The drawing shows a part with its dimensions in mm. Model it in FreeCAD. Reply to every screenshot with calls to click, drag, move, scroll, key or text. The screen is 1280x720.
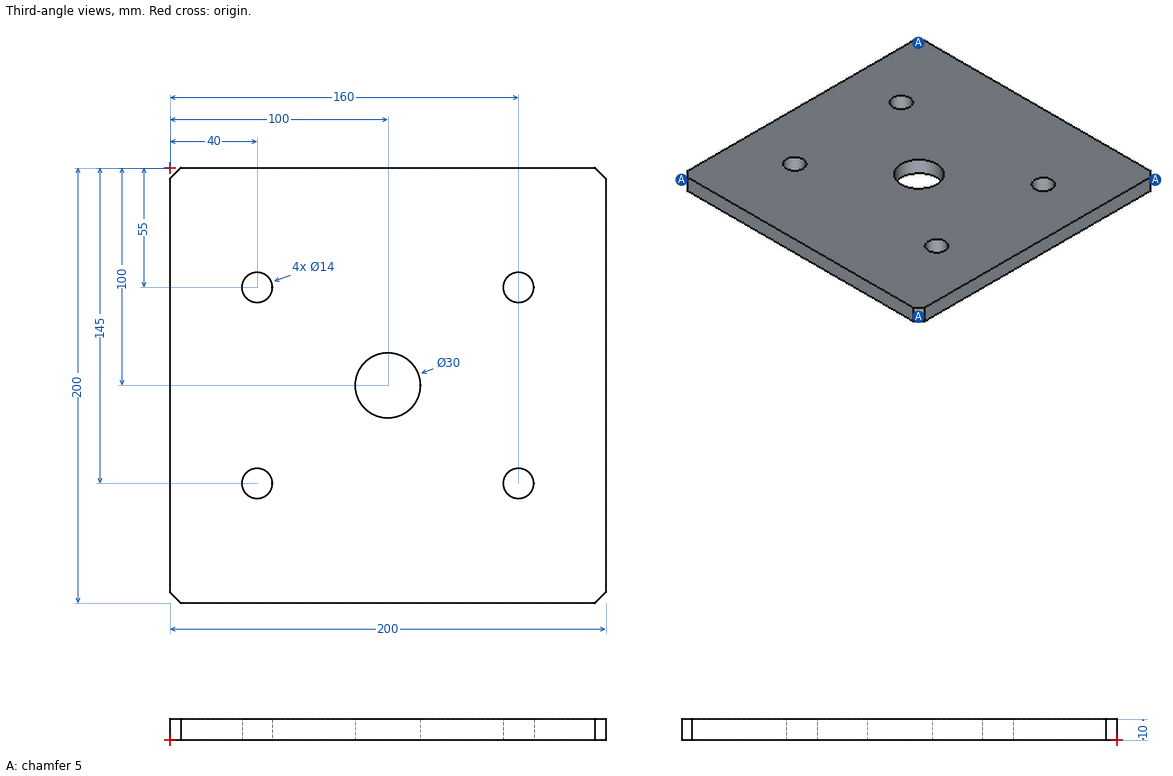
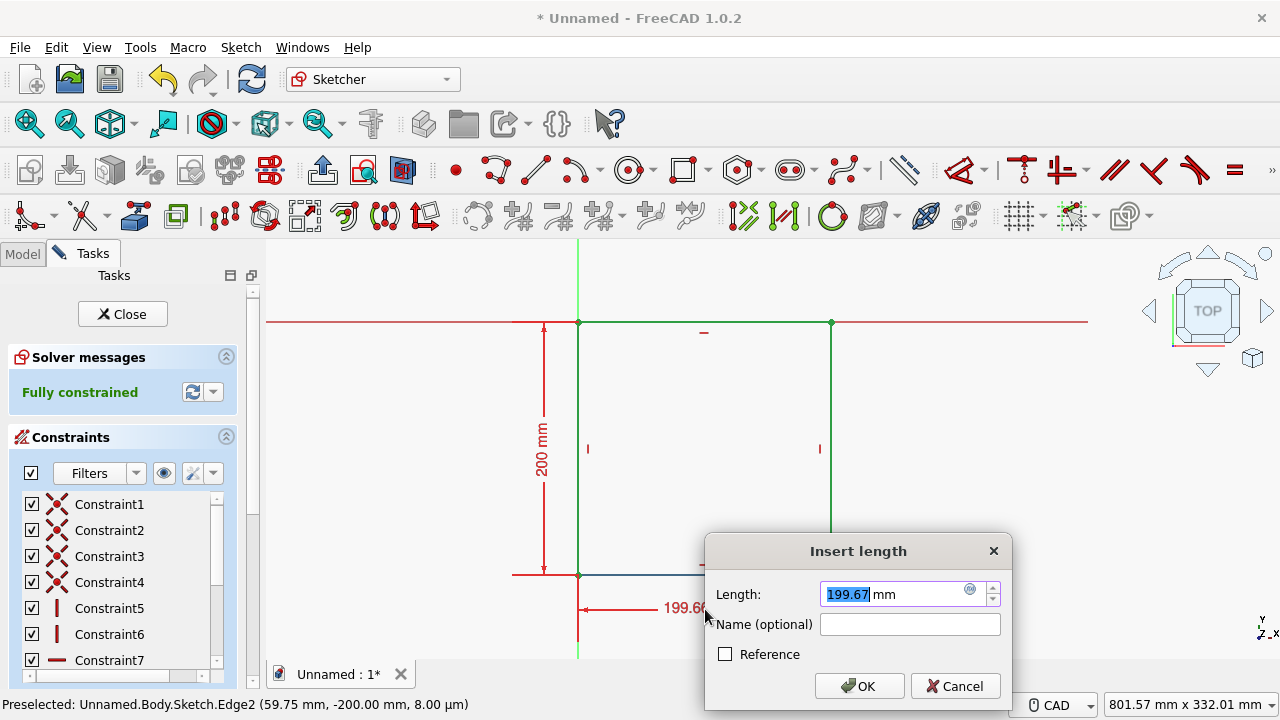
text(200)
key(Return)
key(Escape)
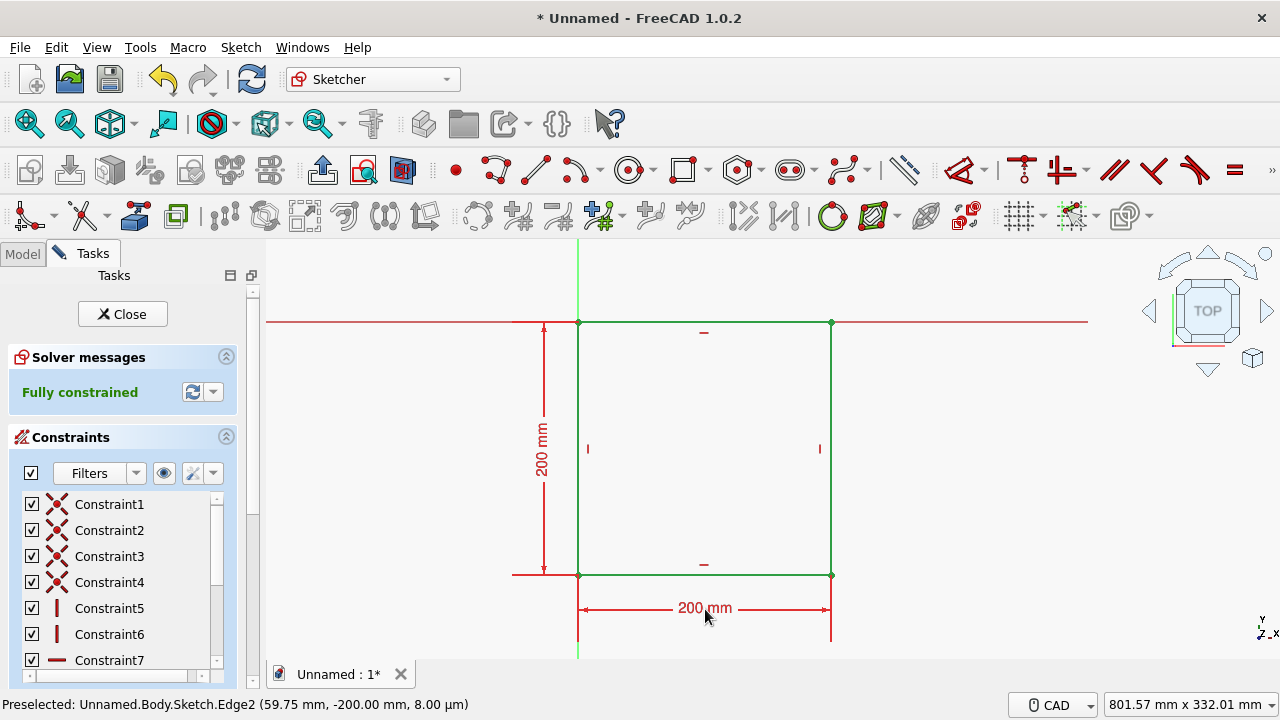
click(123, 314)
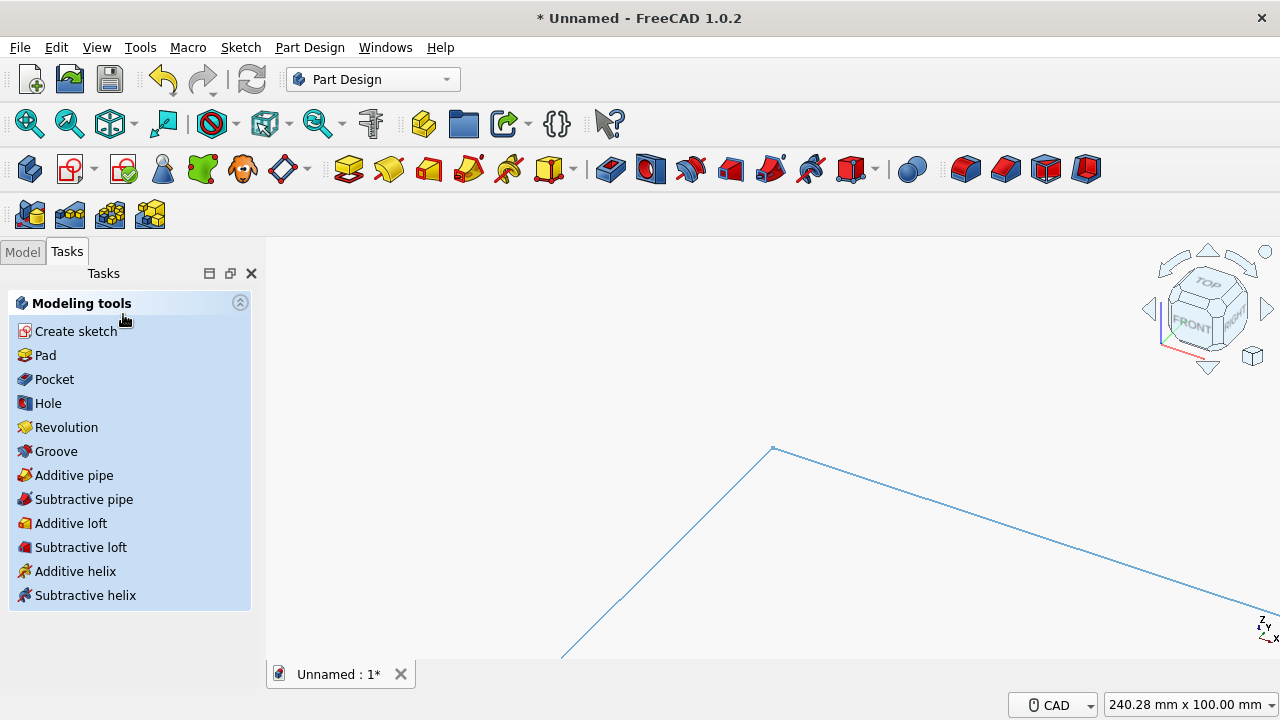
click(350, 170)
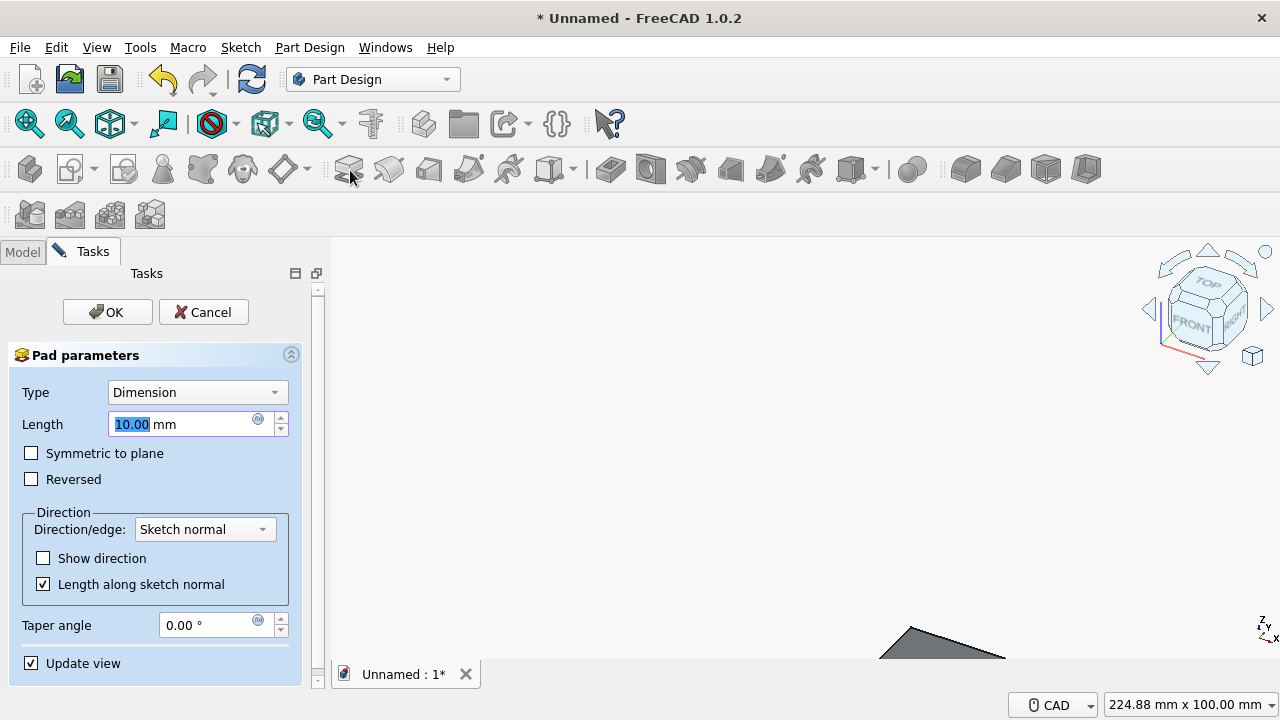
text(10)
key(Tab)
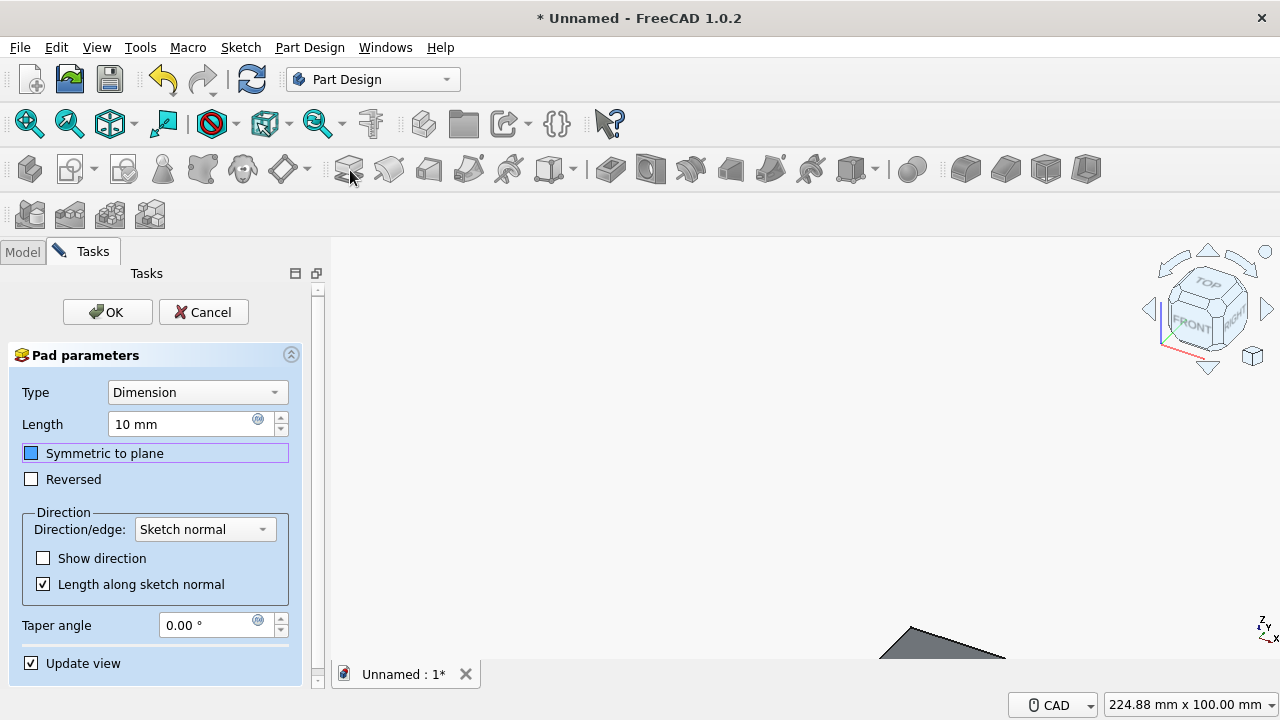
click(108, 312)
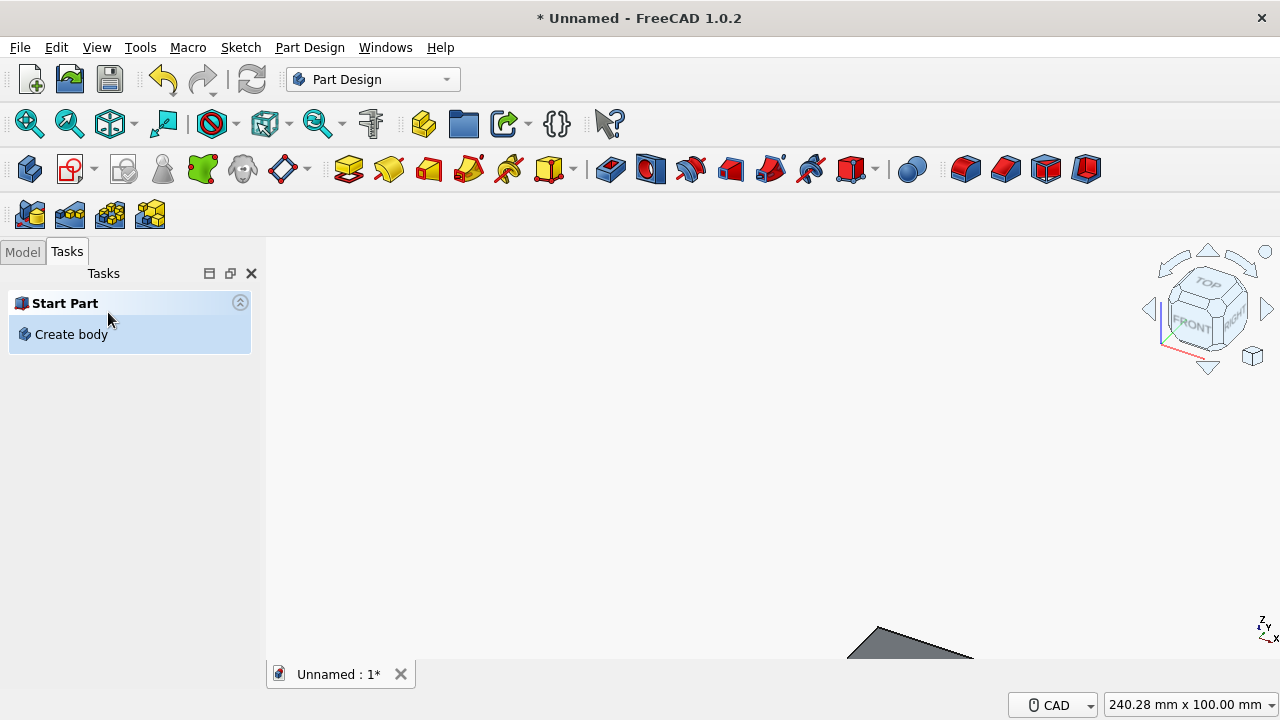
click(30, 124)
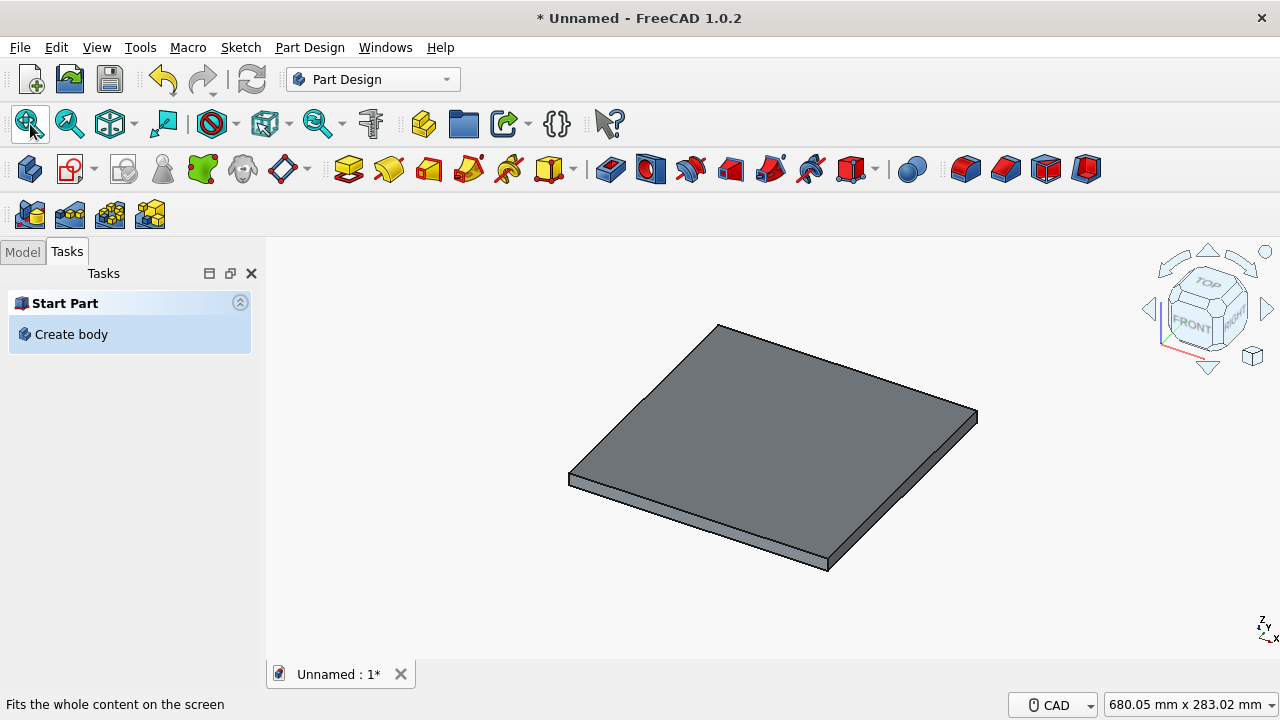
click(773, 441)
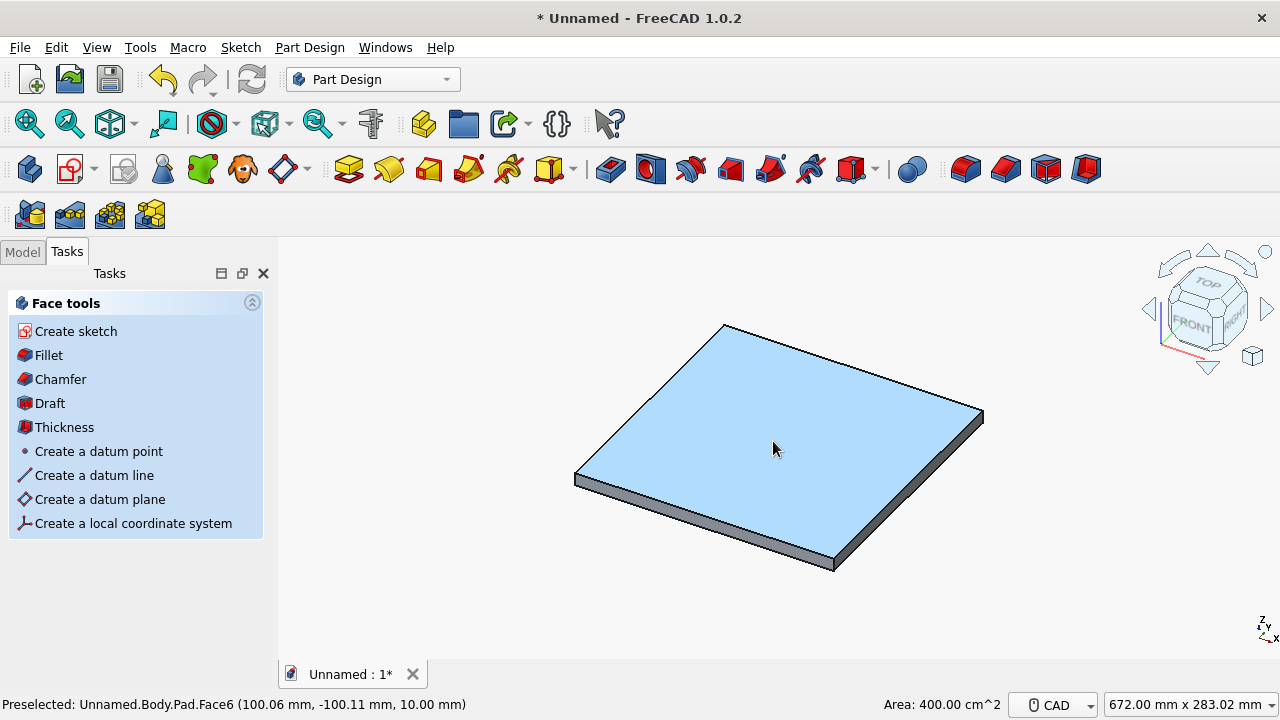
click(70, 170)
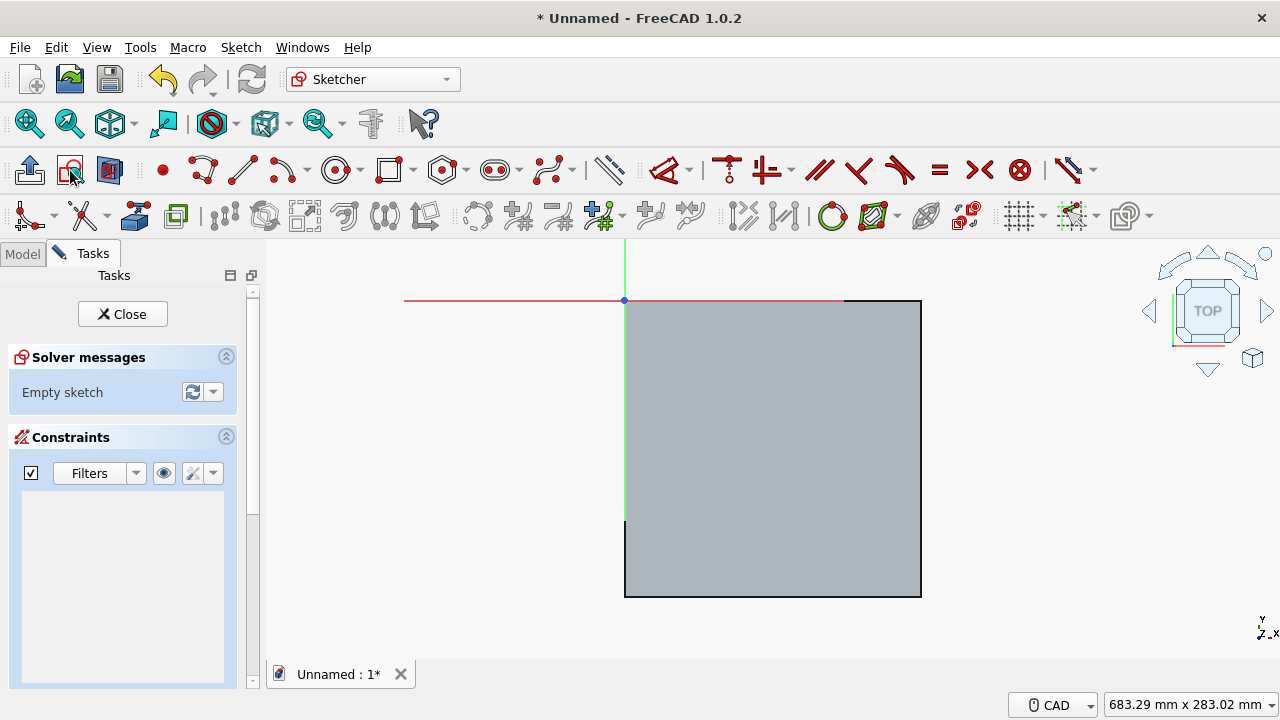
click(336, 170)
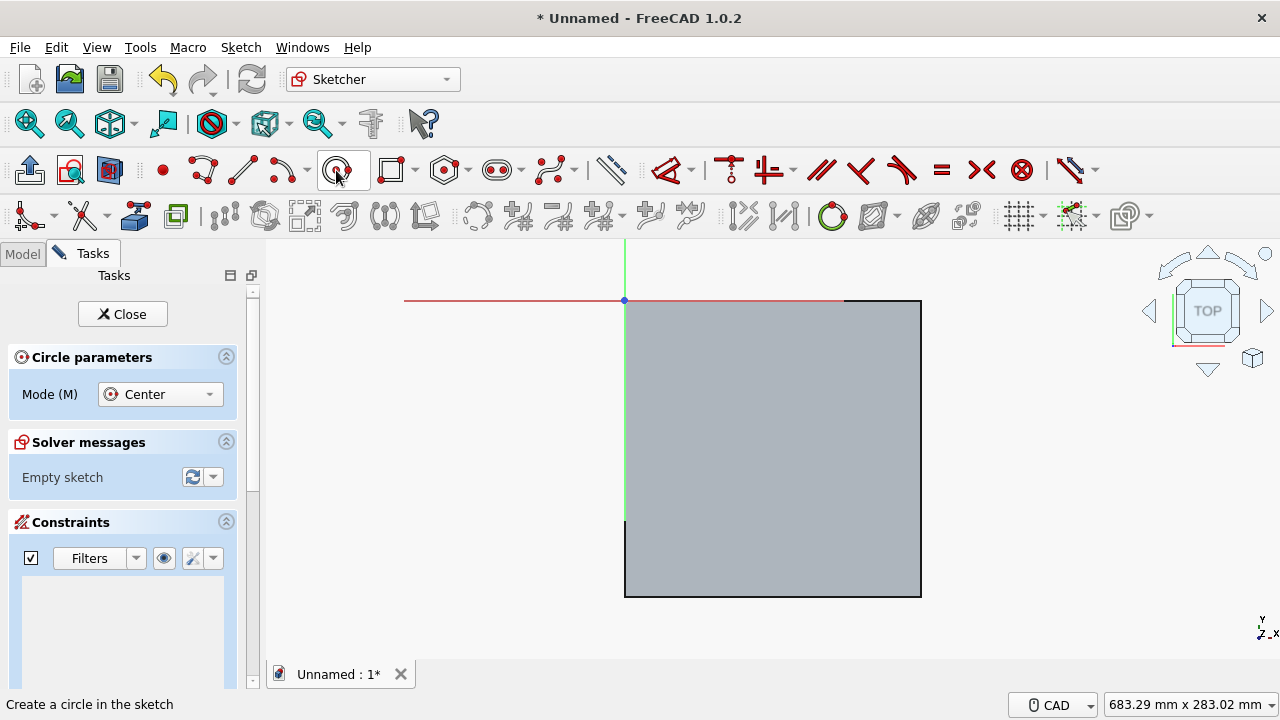
scroll(684, 382, up, 4)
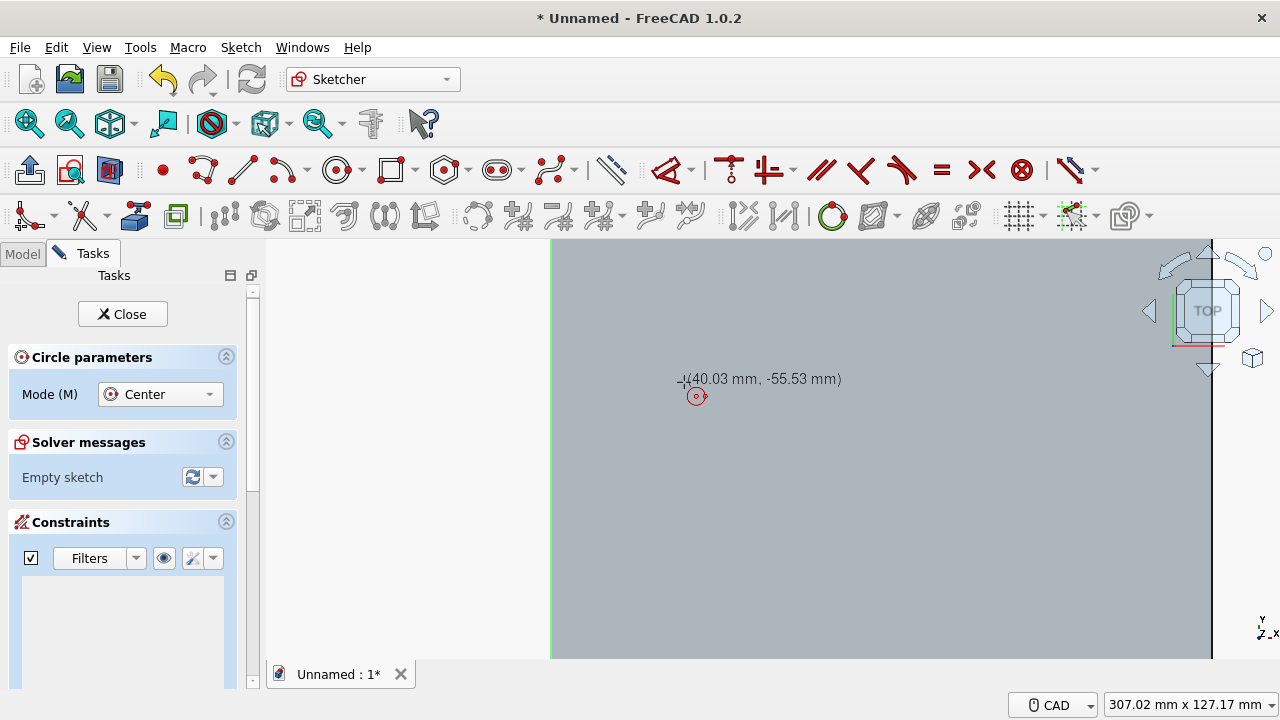
click(683, 382)
click(700, 366)